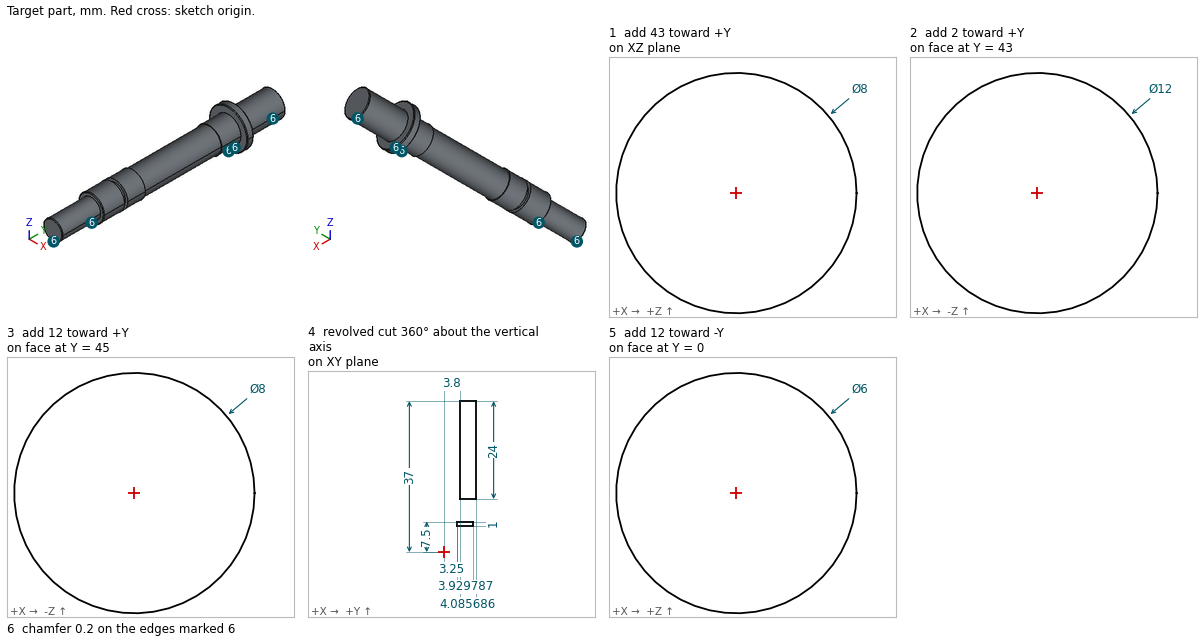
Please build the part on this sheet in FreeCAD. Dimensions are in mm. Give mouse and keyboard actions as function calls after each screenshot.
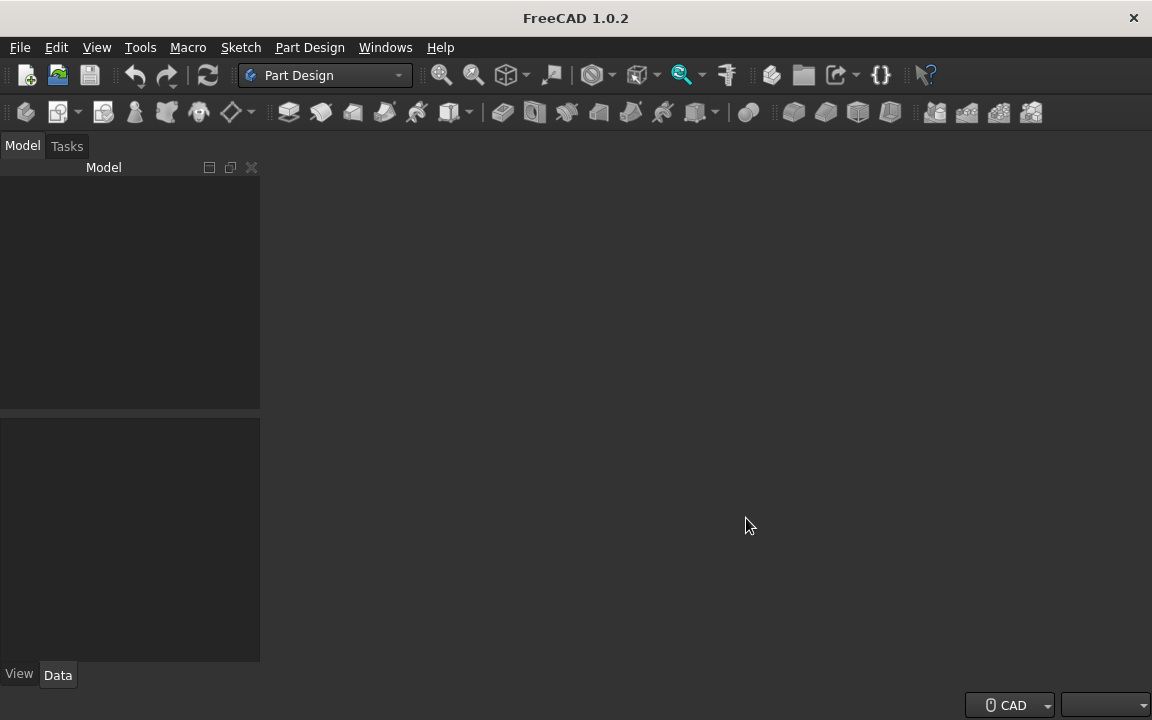
click(26, 76)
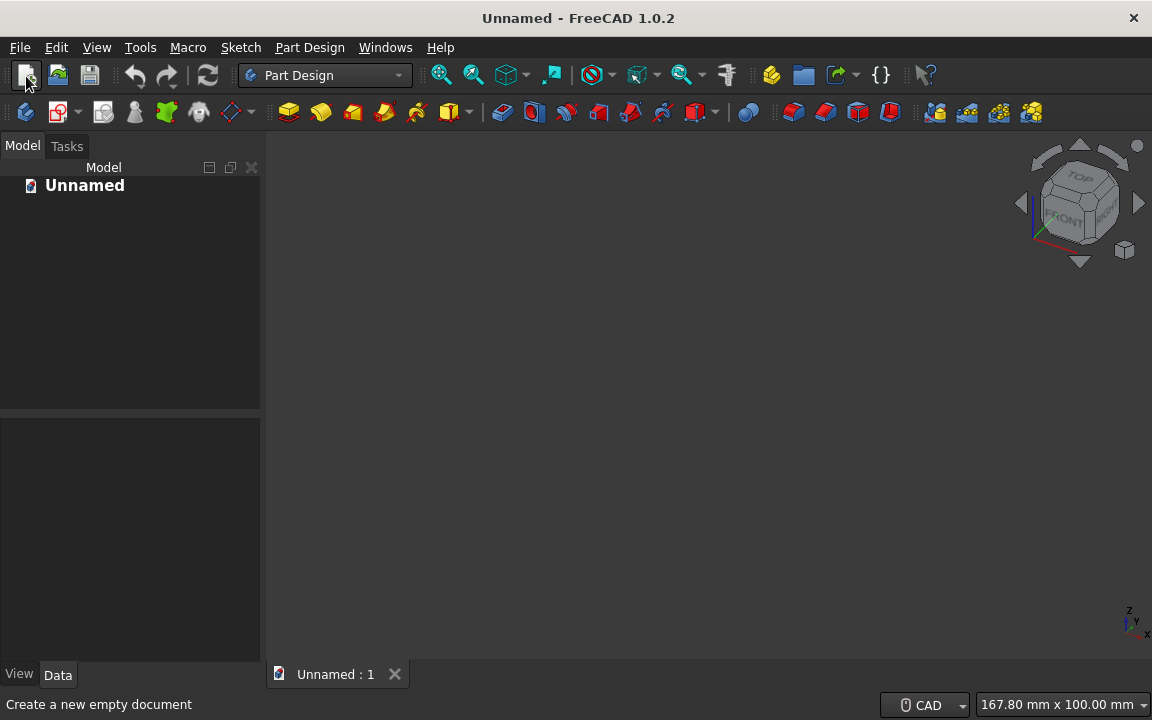
click(58, 112)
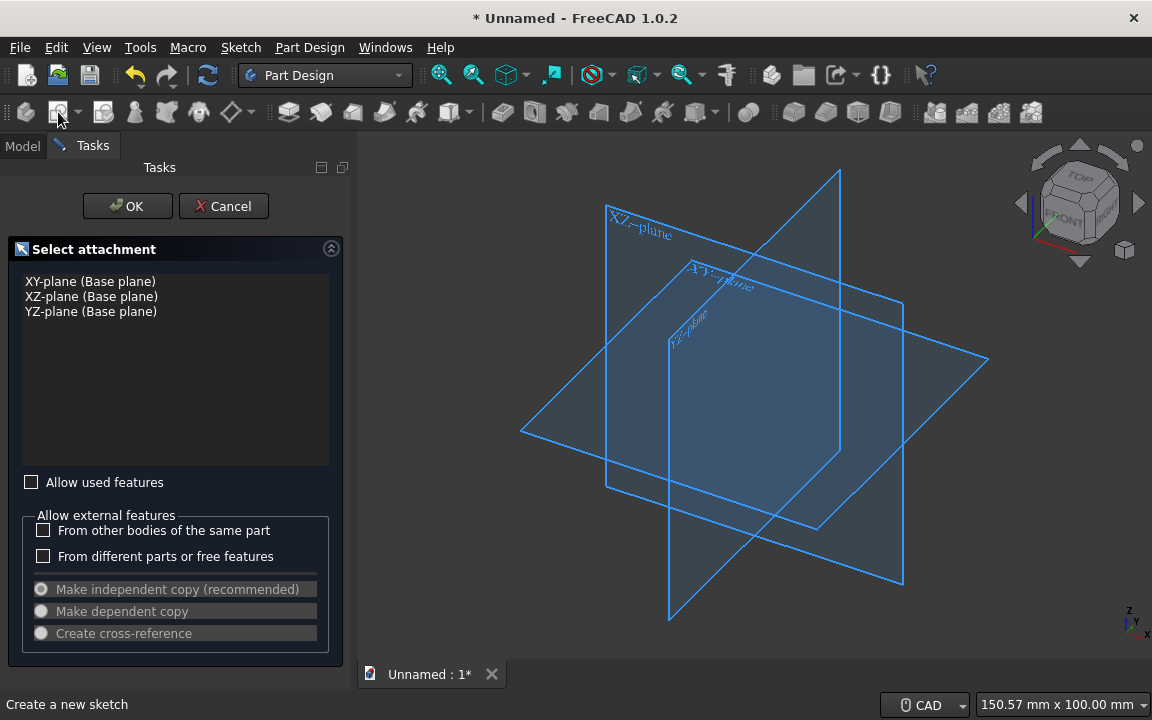
click(82, 296)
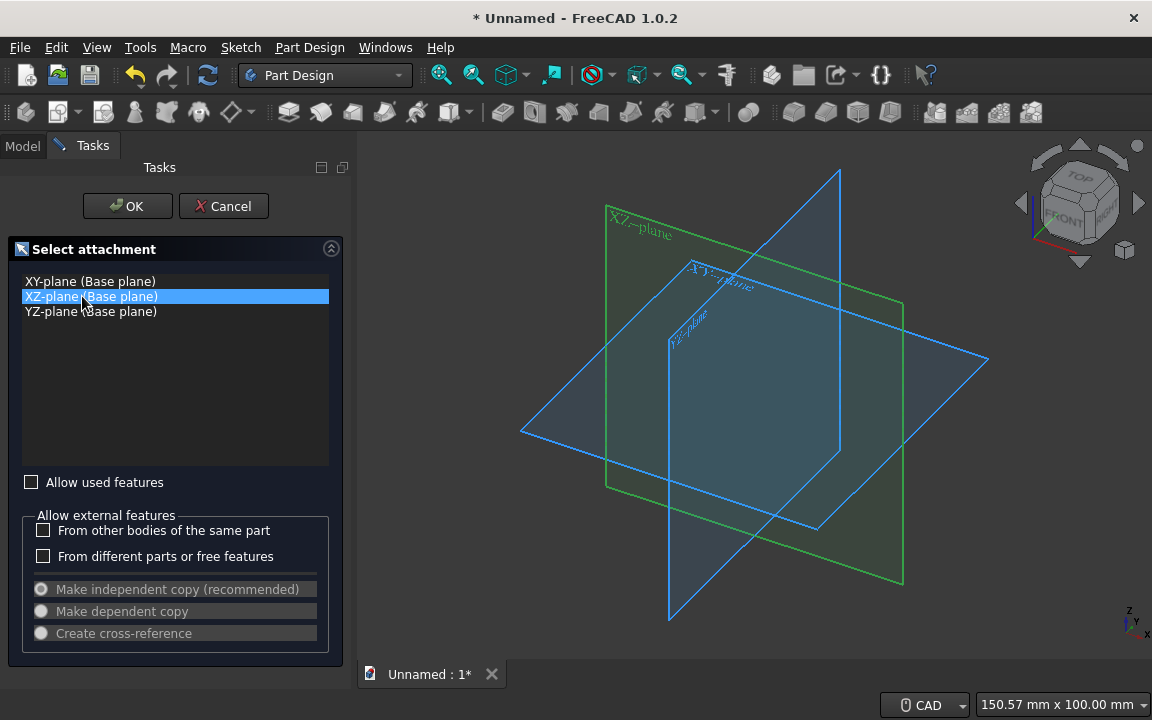
click(128, 206)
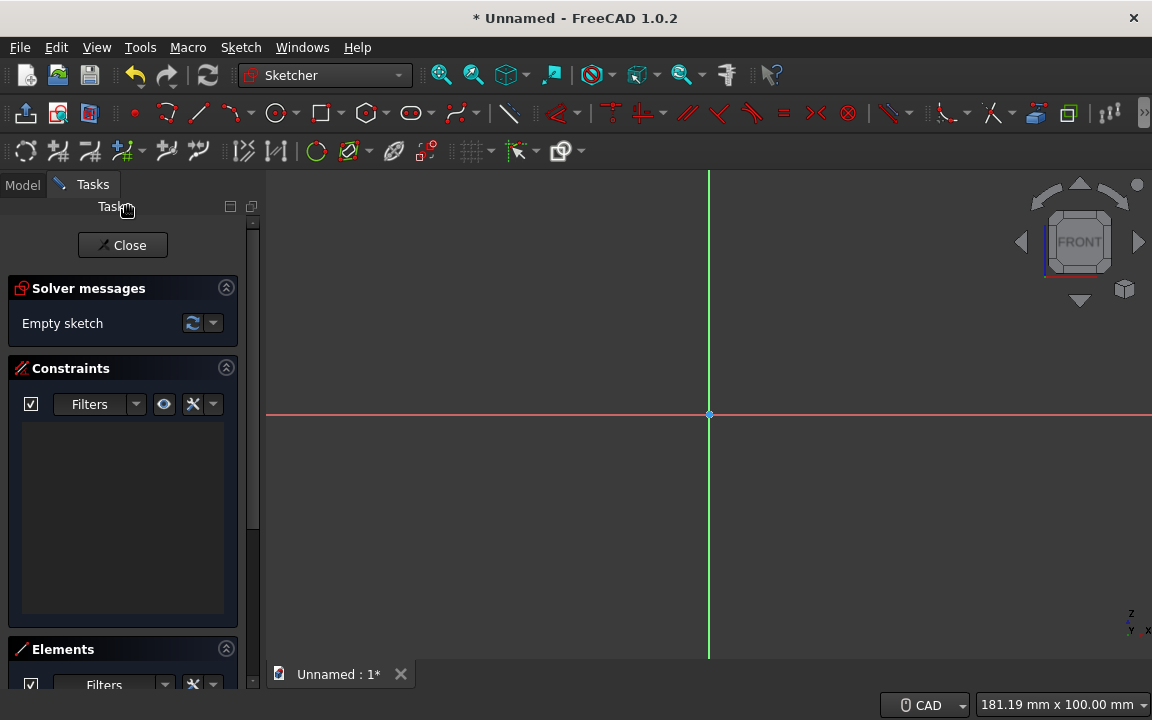
scroll(720, 414, up, 10)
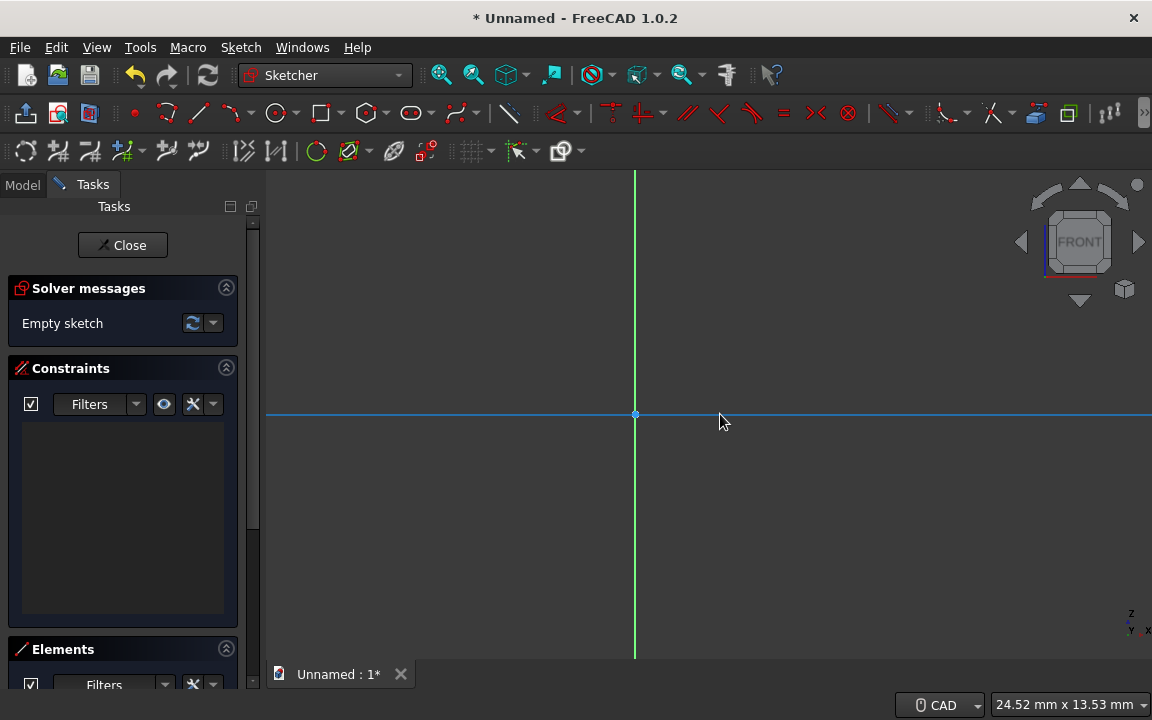
click(276, 114)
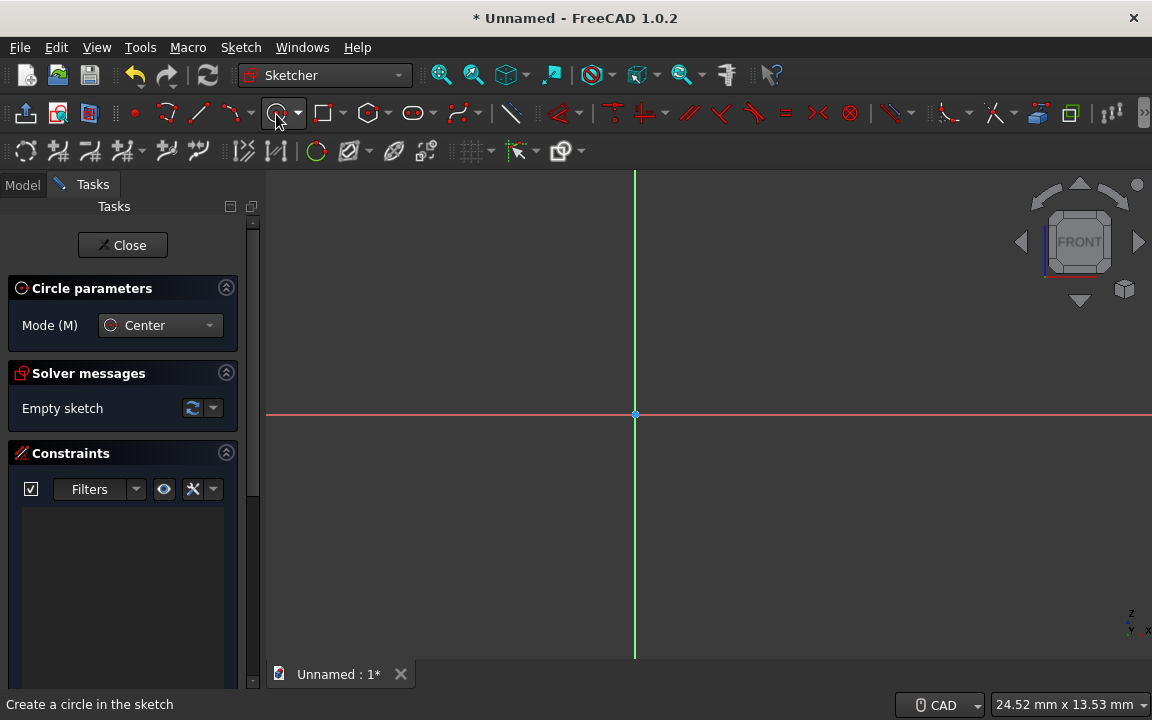
click(635, 414)
move(738, 312)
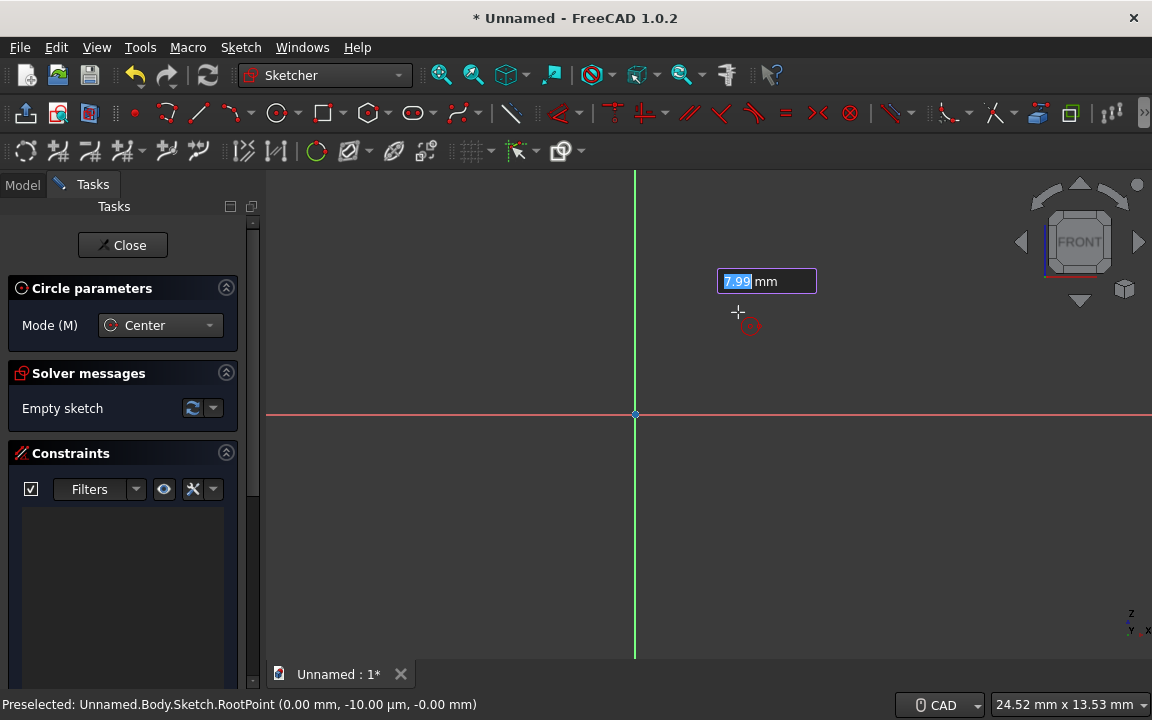
text(8)
key(Return)
key(Escape)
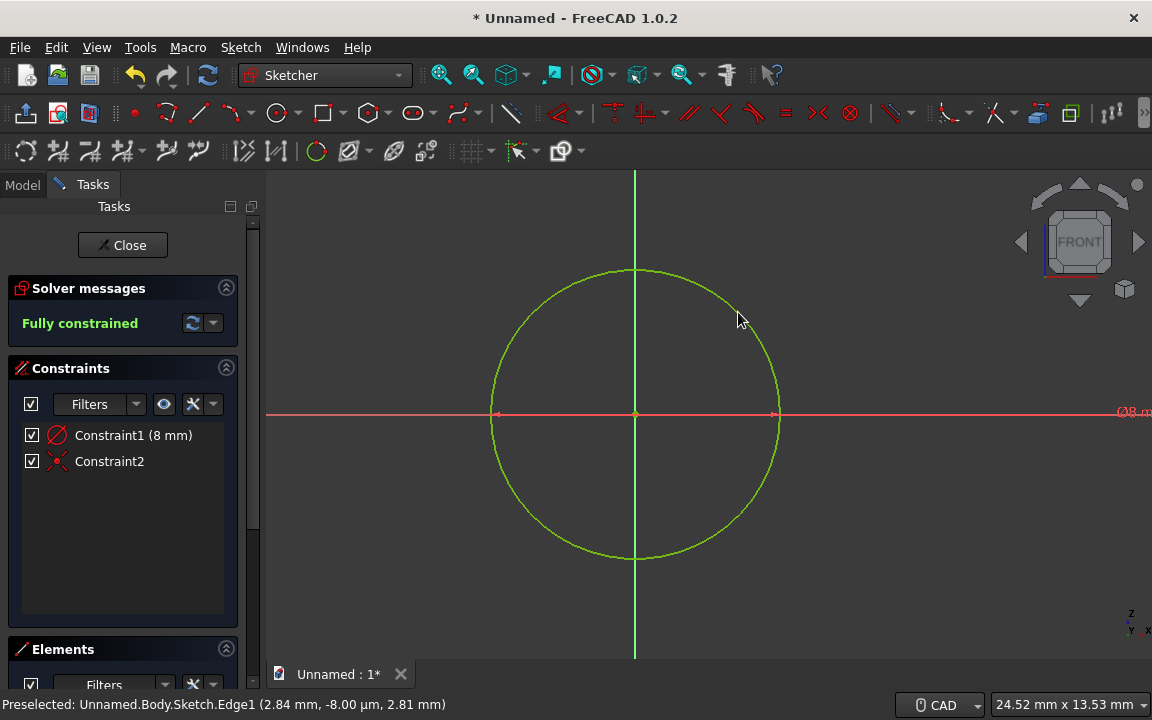
click(123, 245)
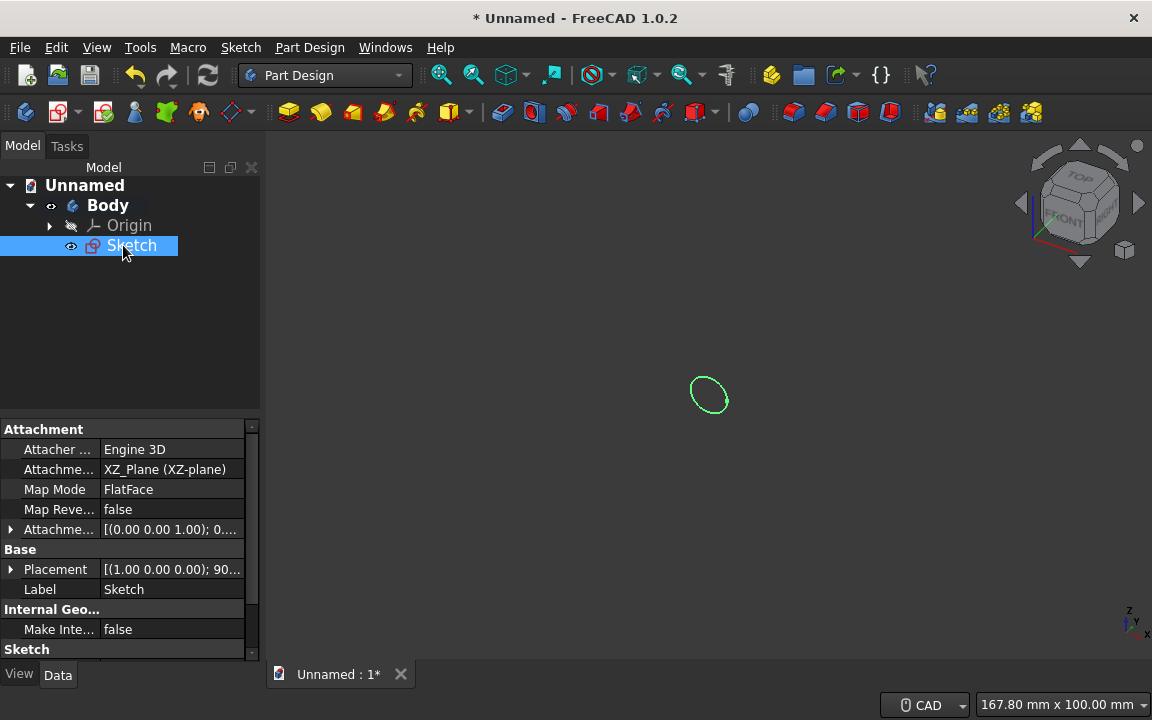
click(290, 112)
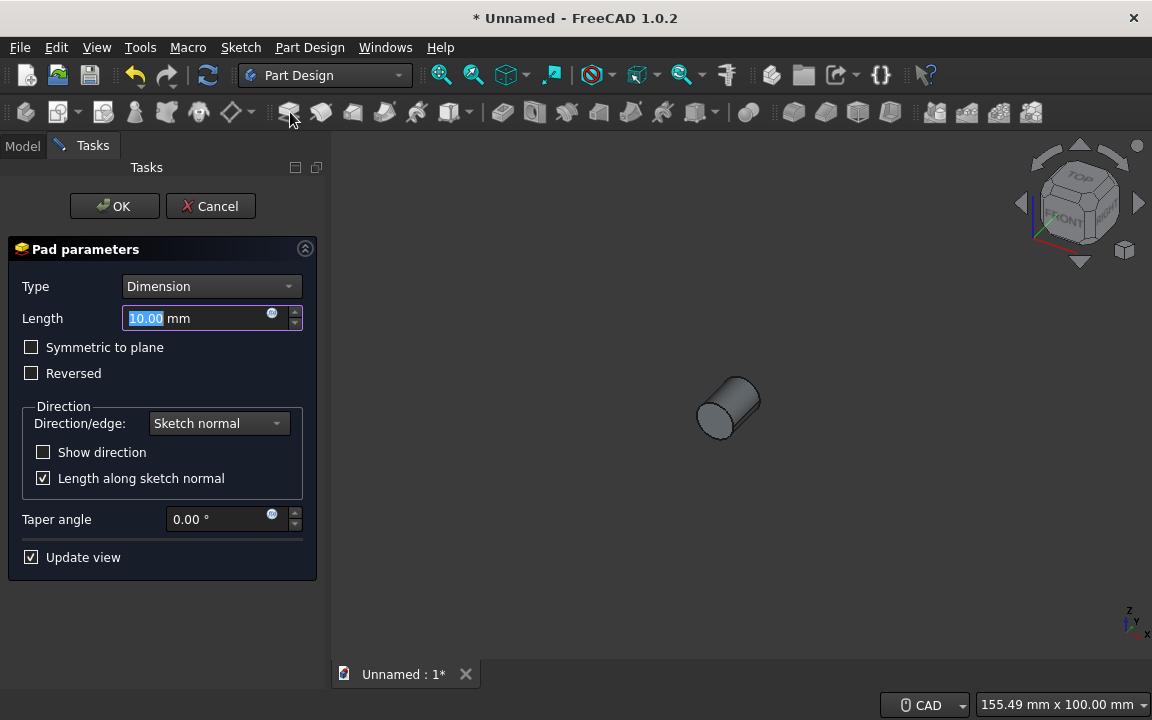
text(43)
key(Tab)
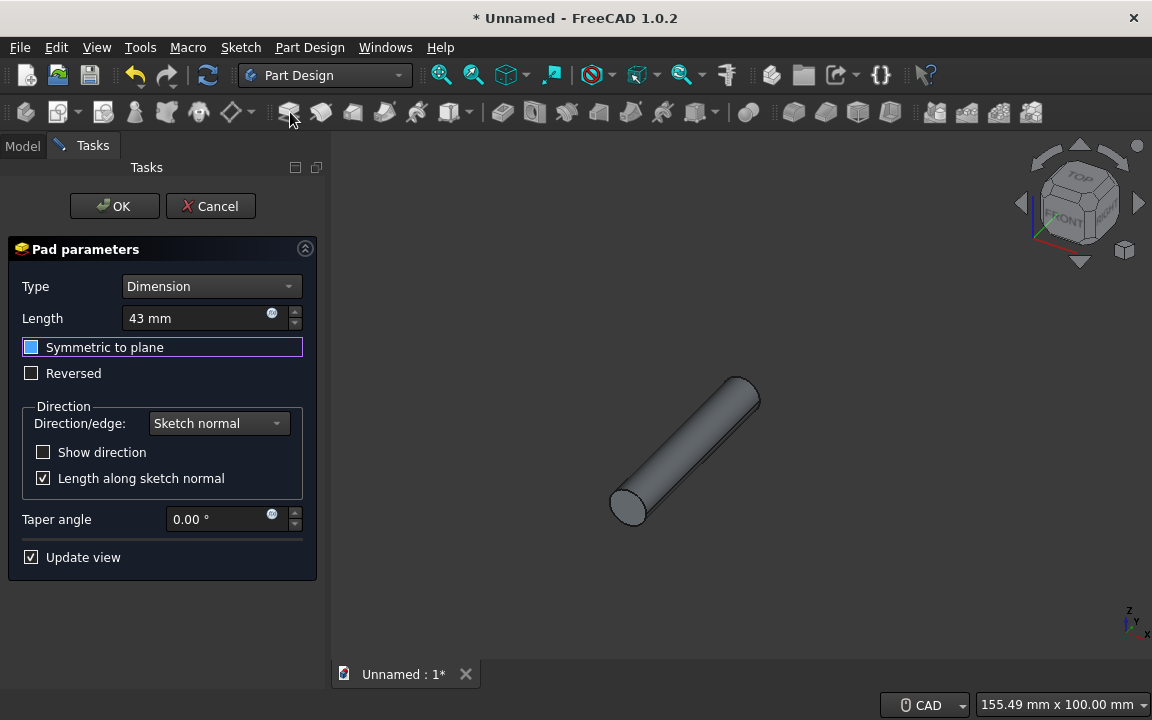
click(30, 373)